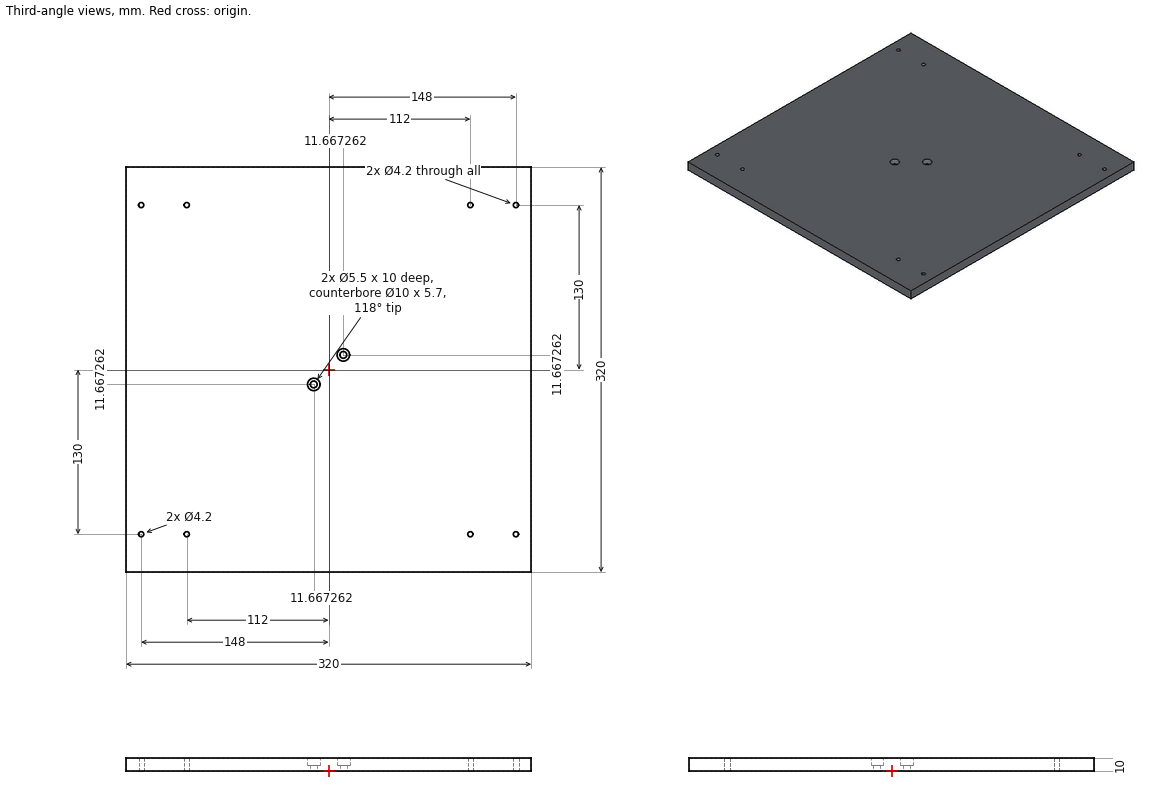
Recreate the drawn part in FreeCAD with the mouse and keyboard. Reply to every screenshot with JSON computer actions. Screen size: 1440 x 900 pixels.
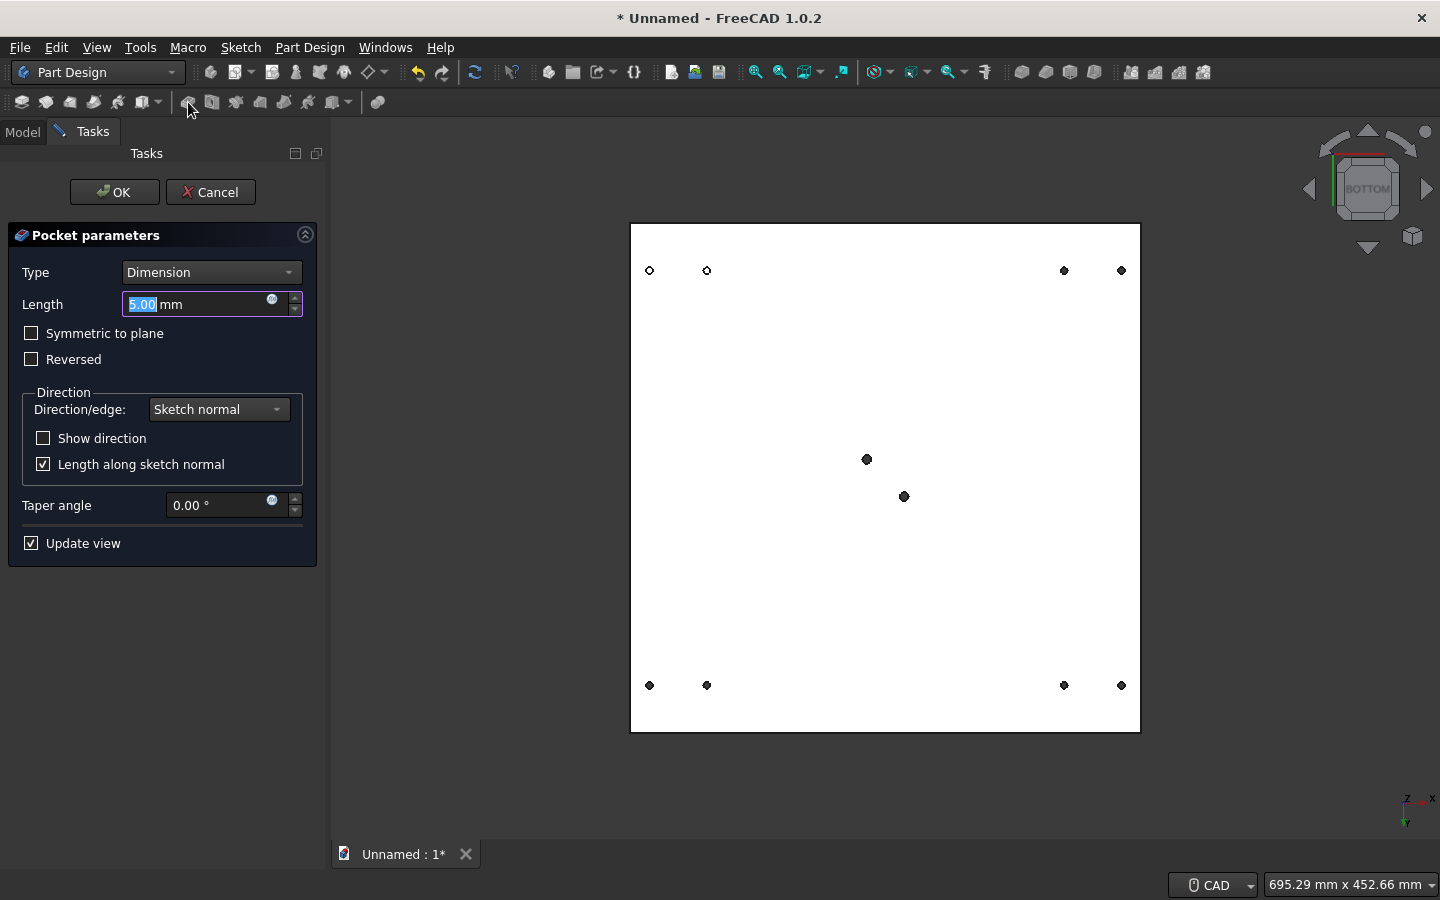
{"action": "left_click", "coordinate": [212, 272]}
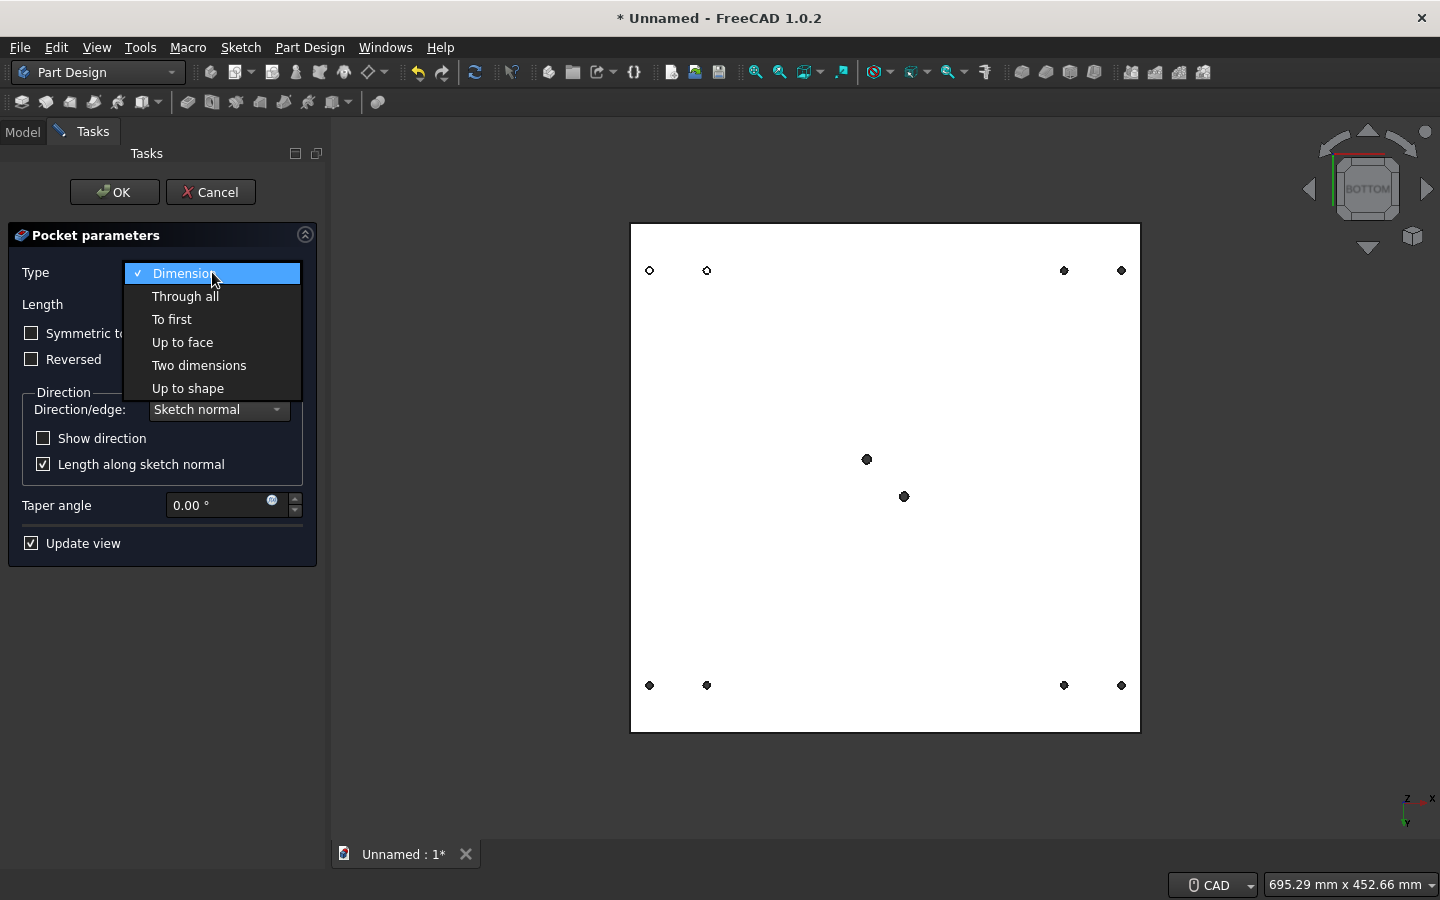
{"action": "left_click", "coordinate": [212, 296]}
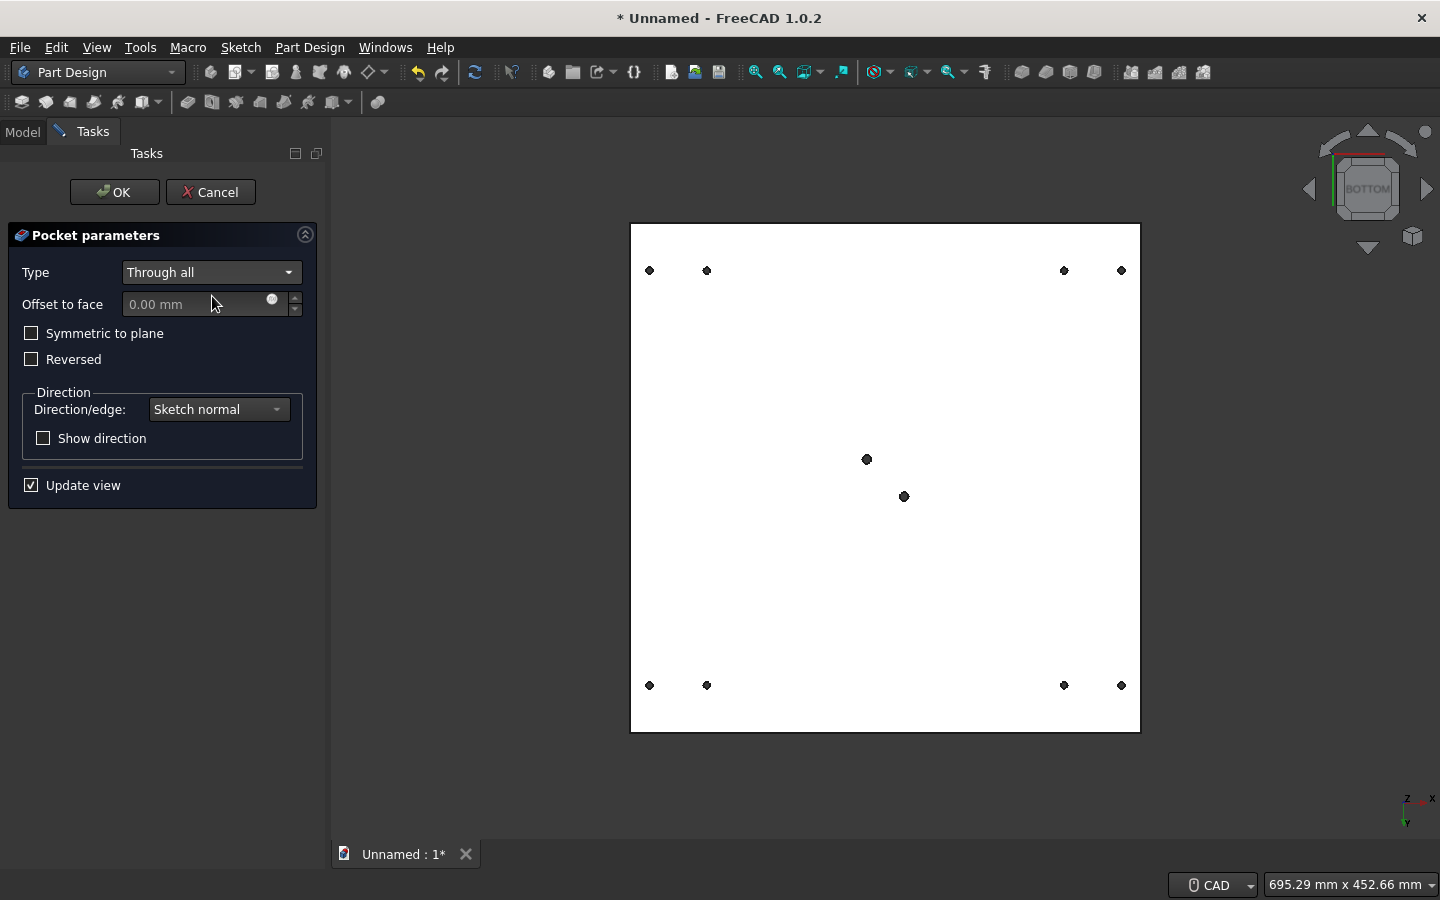
{"action": "left_click", "coordinate": [115, 192]}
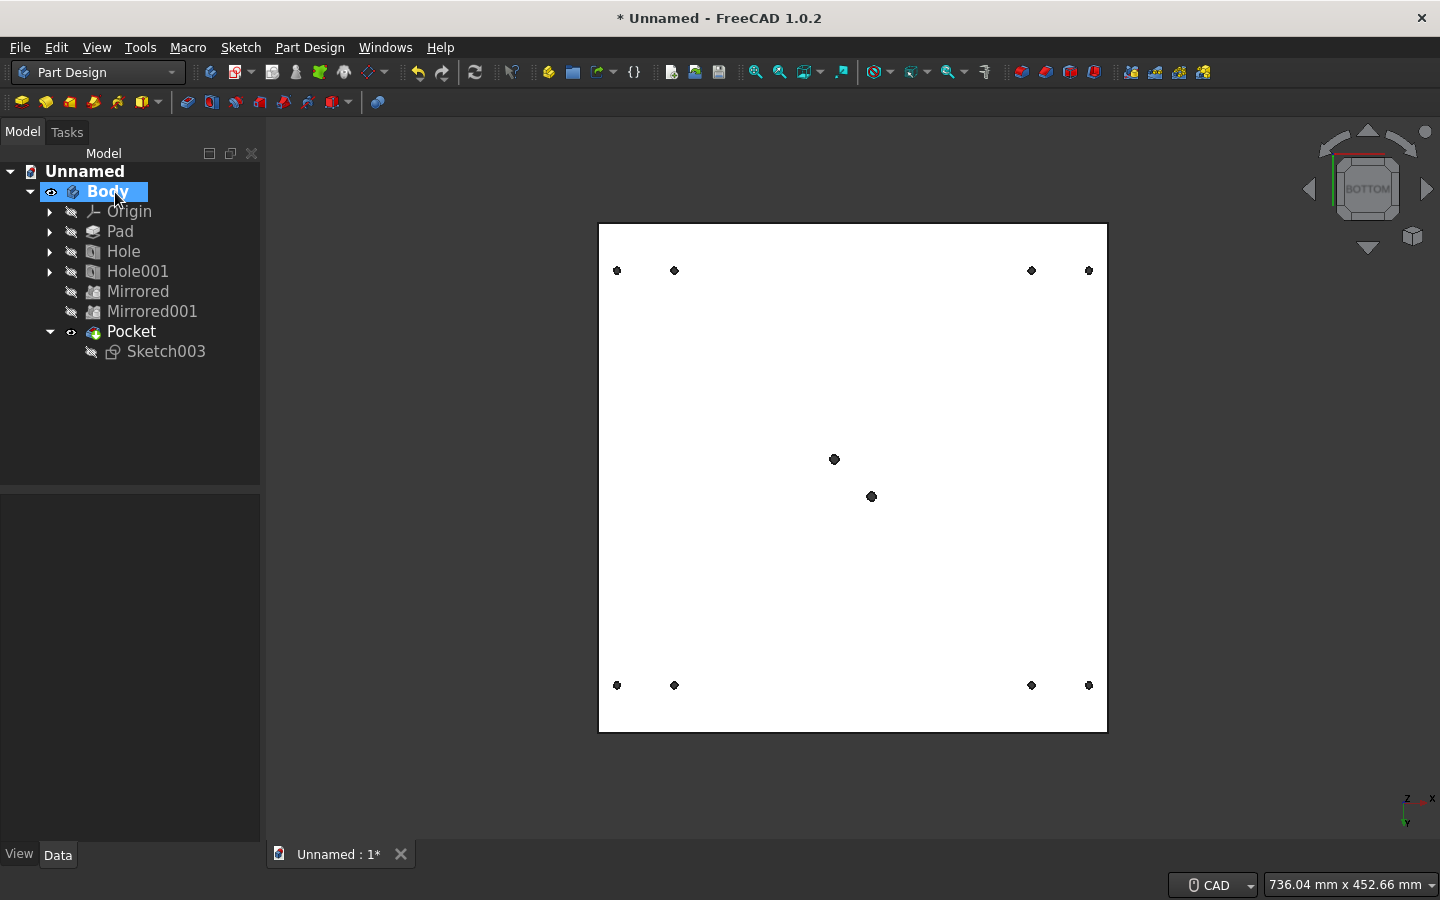
{"action": "key", "text": "0"}